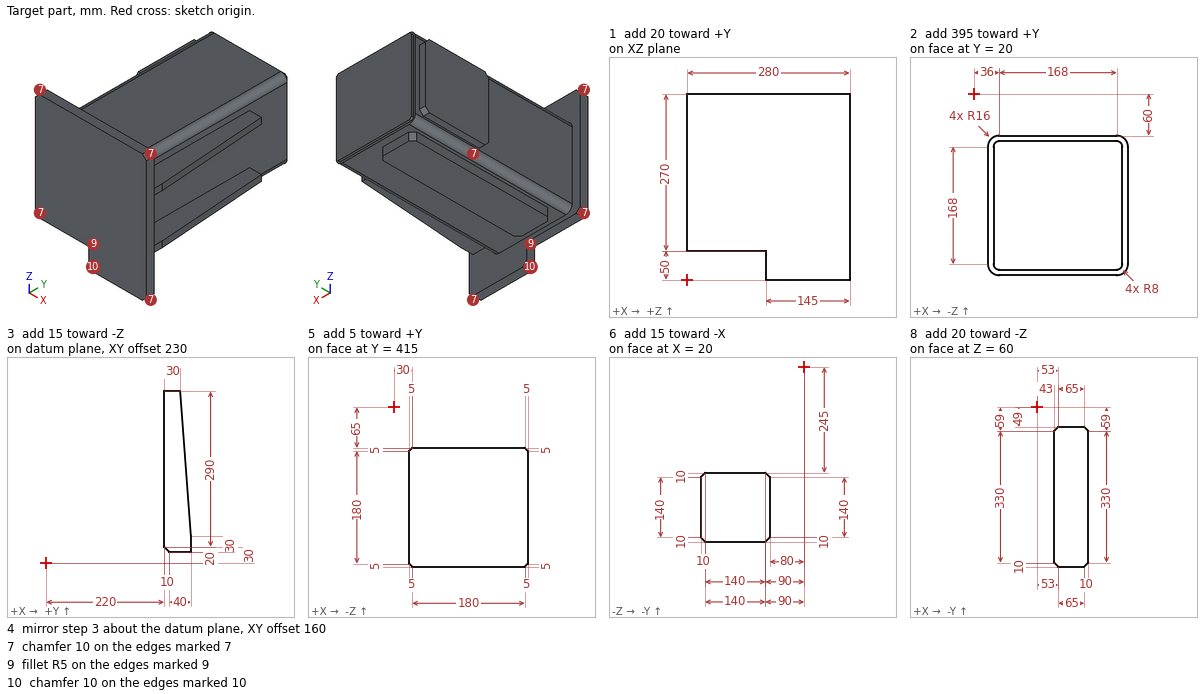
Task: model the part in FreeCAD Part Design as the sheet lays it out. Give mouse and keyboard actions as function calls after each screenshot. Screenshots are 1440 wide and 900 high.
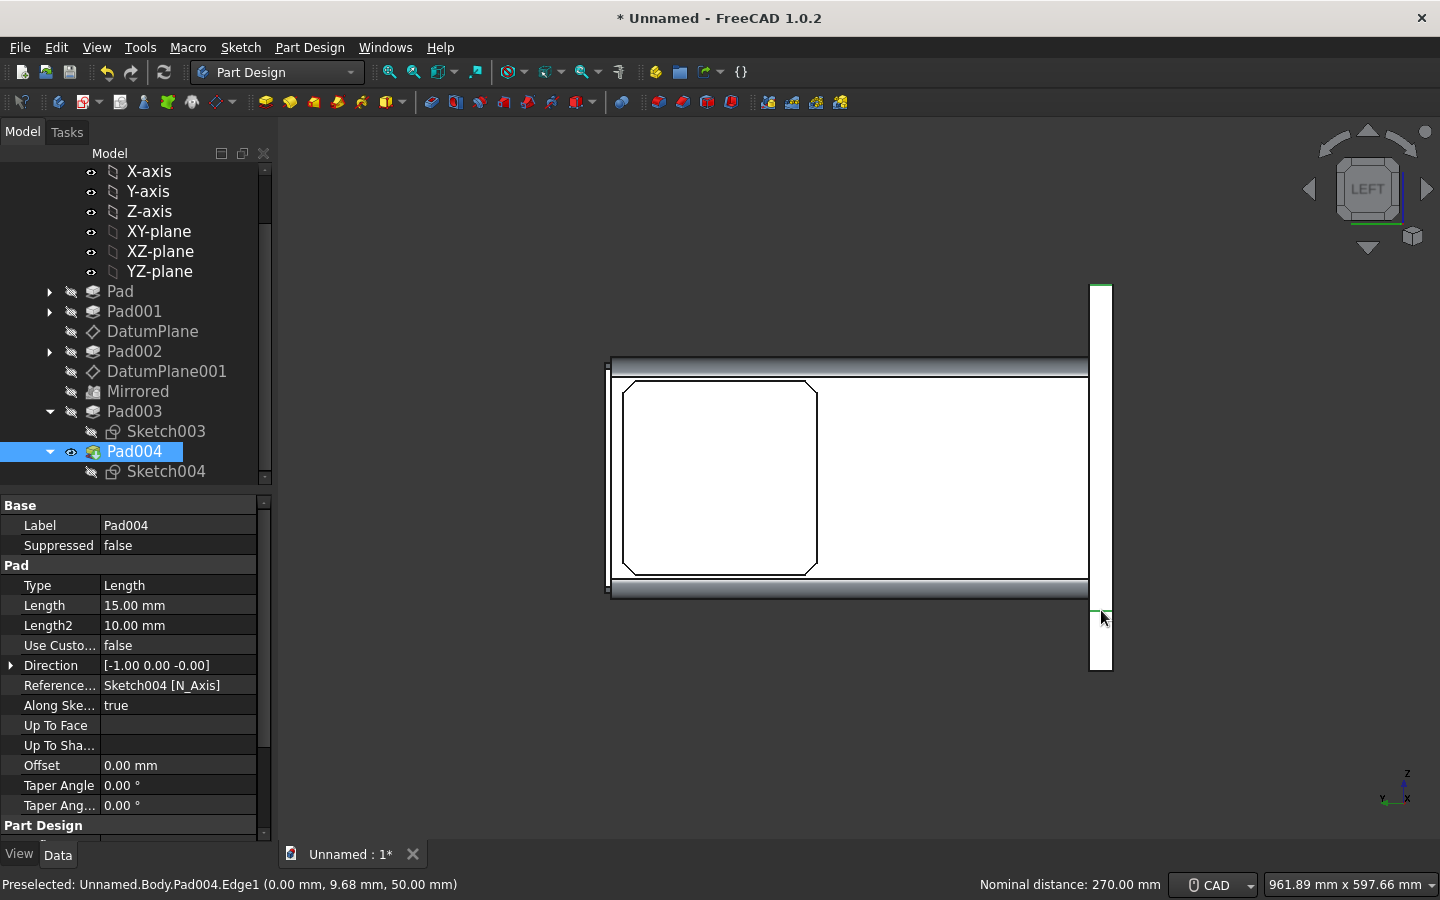
key(0)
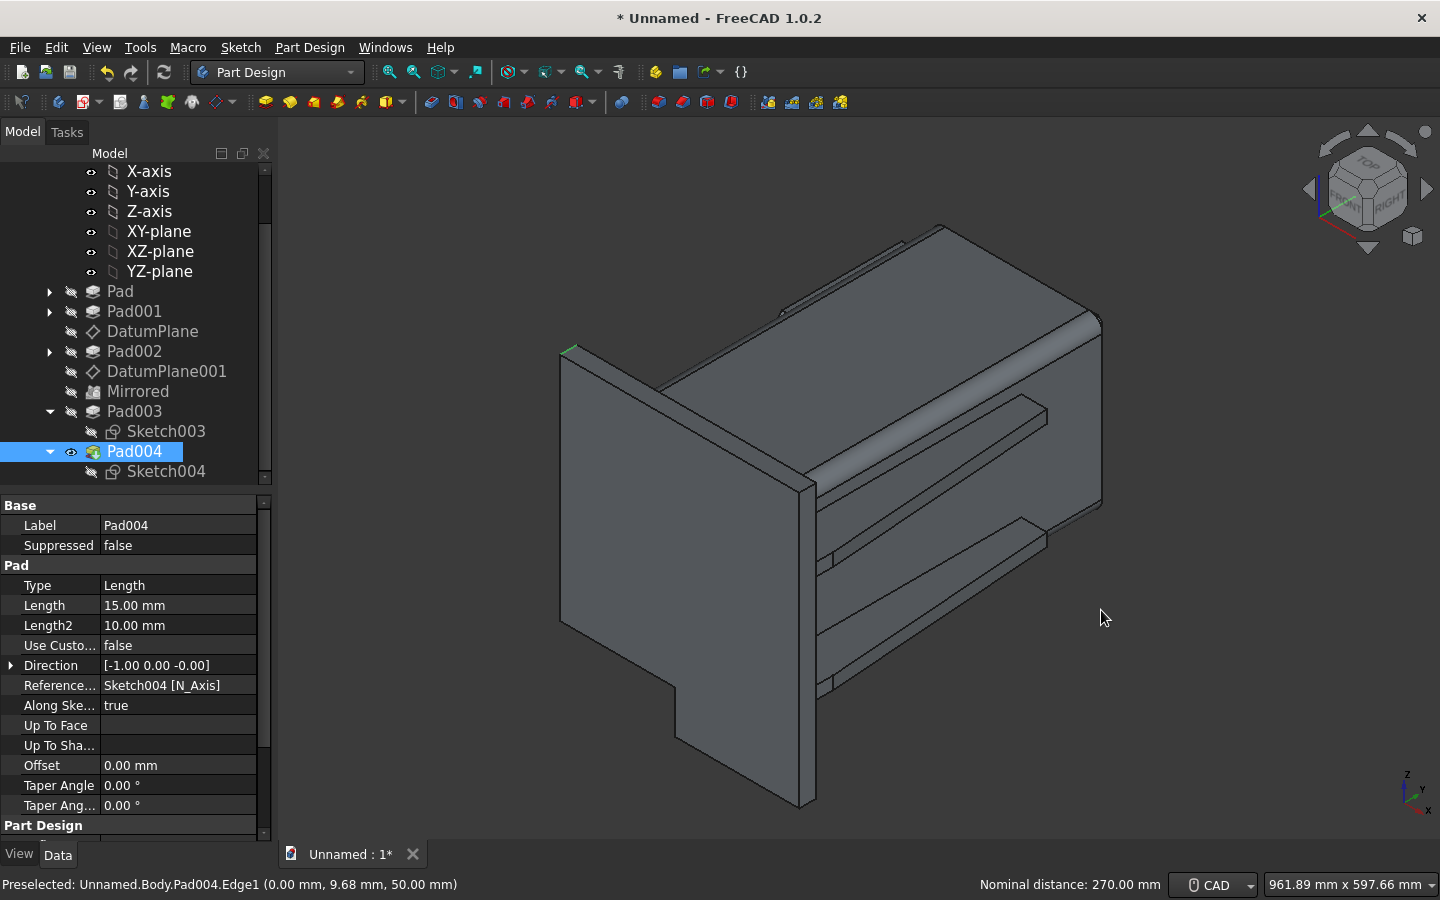
click(808, 487, ctrl)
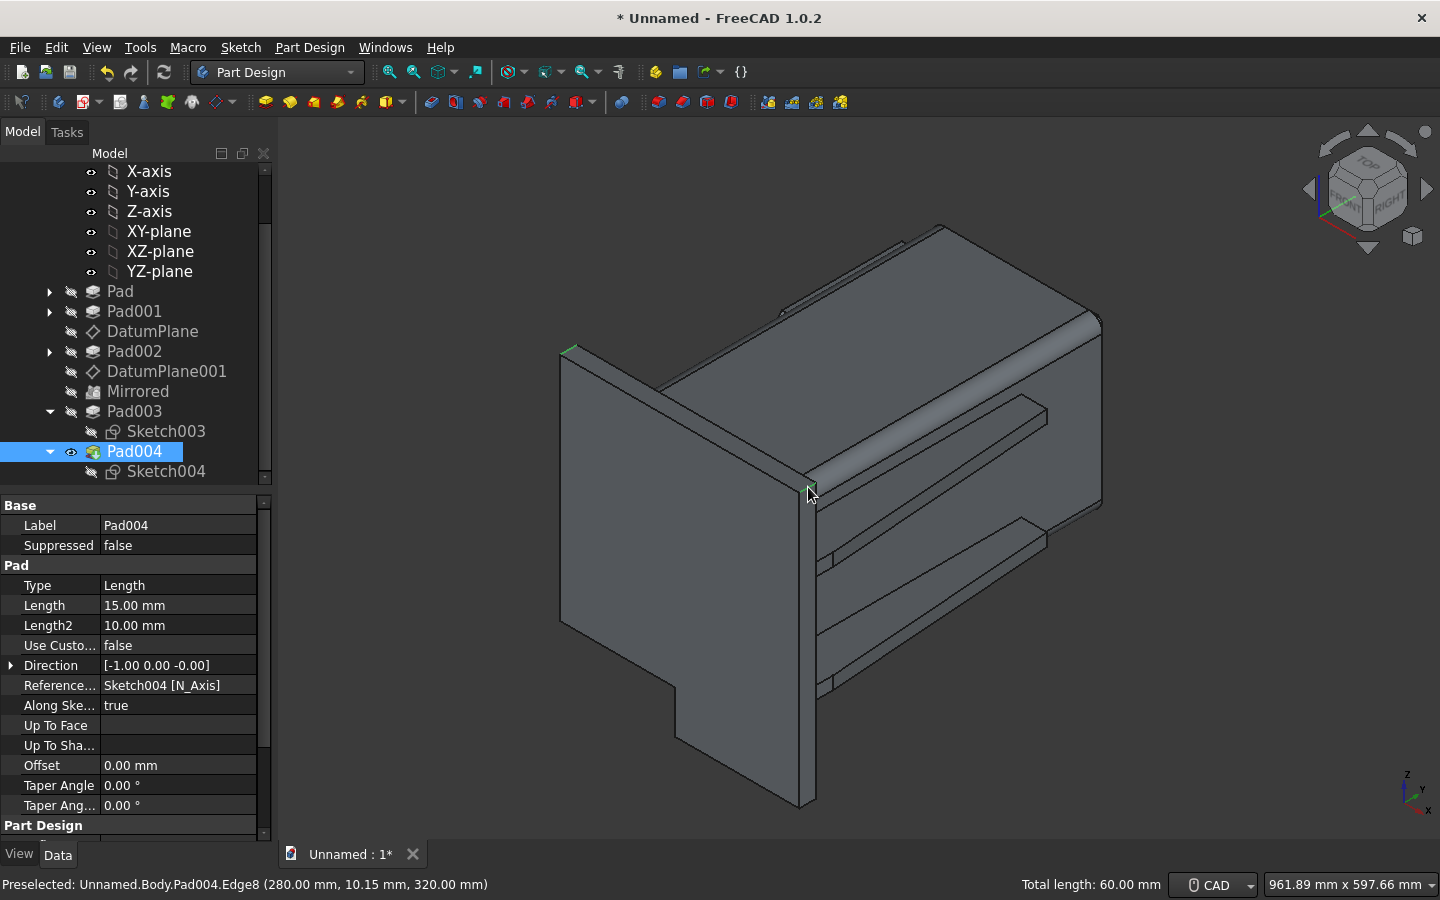
key(2)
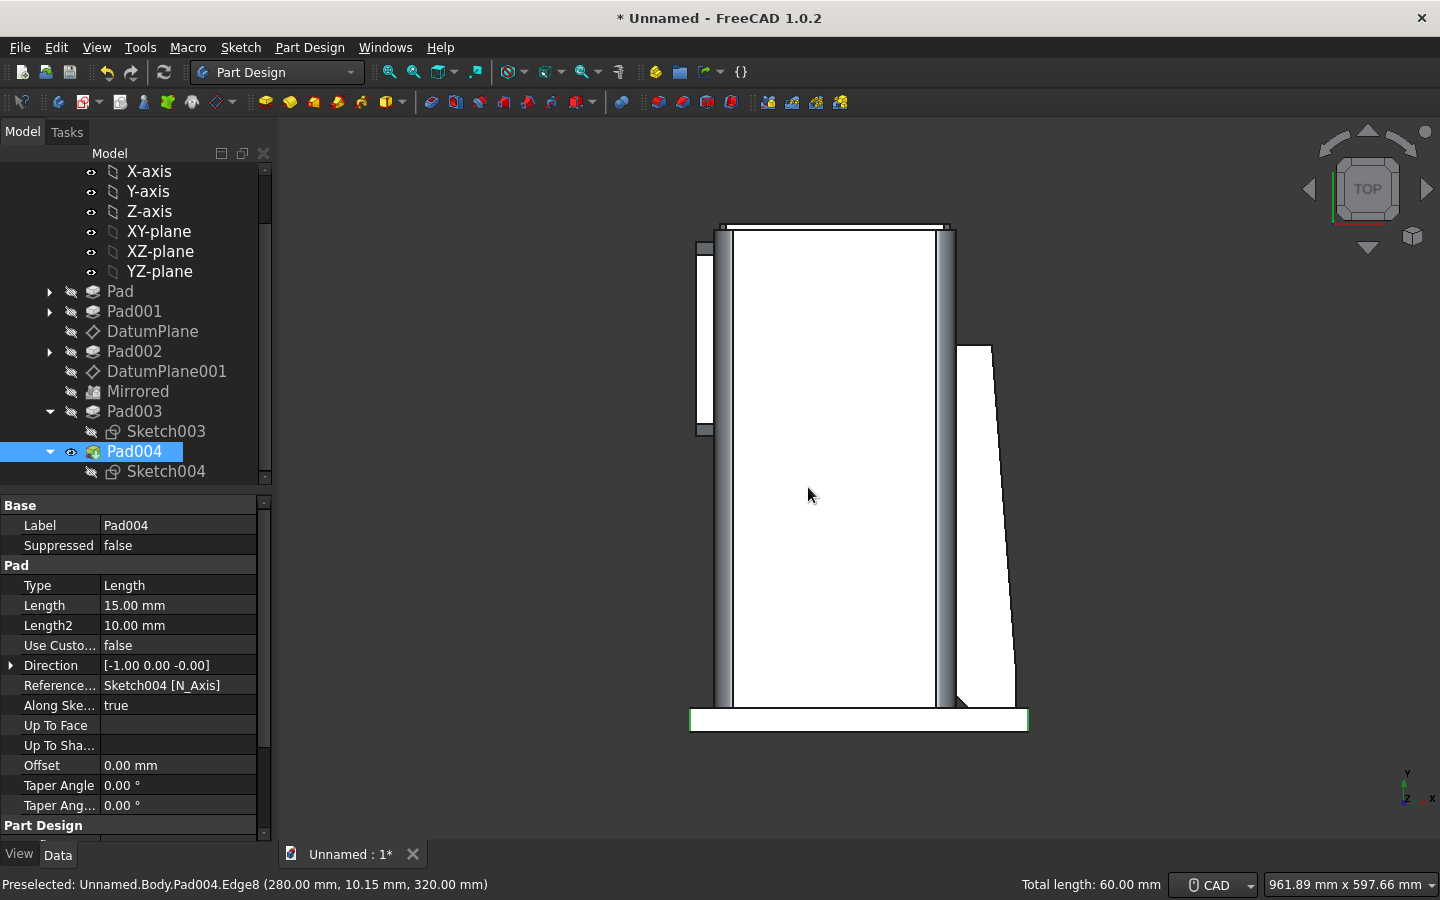
key(1)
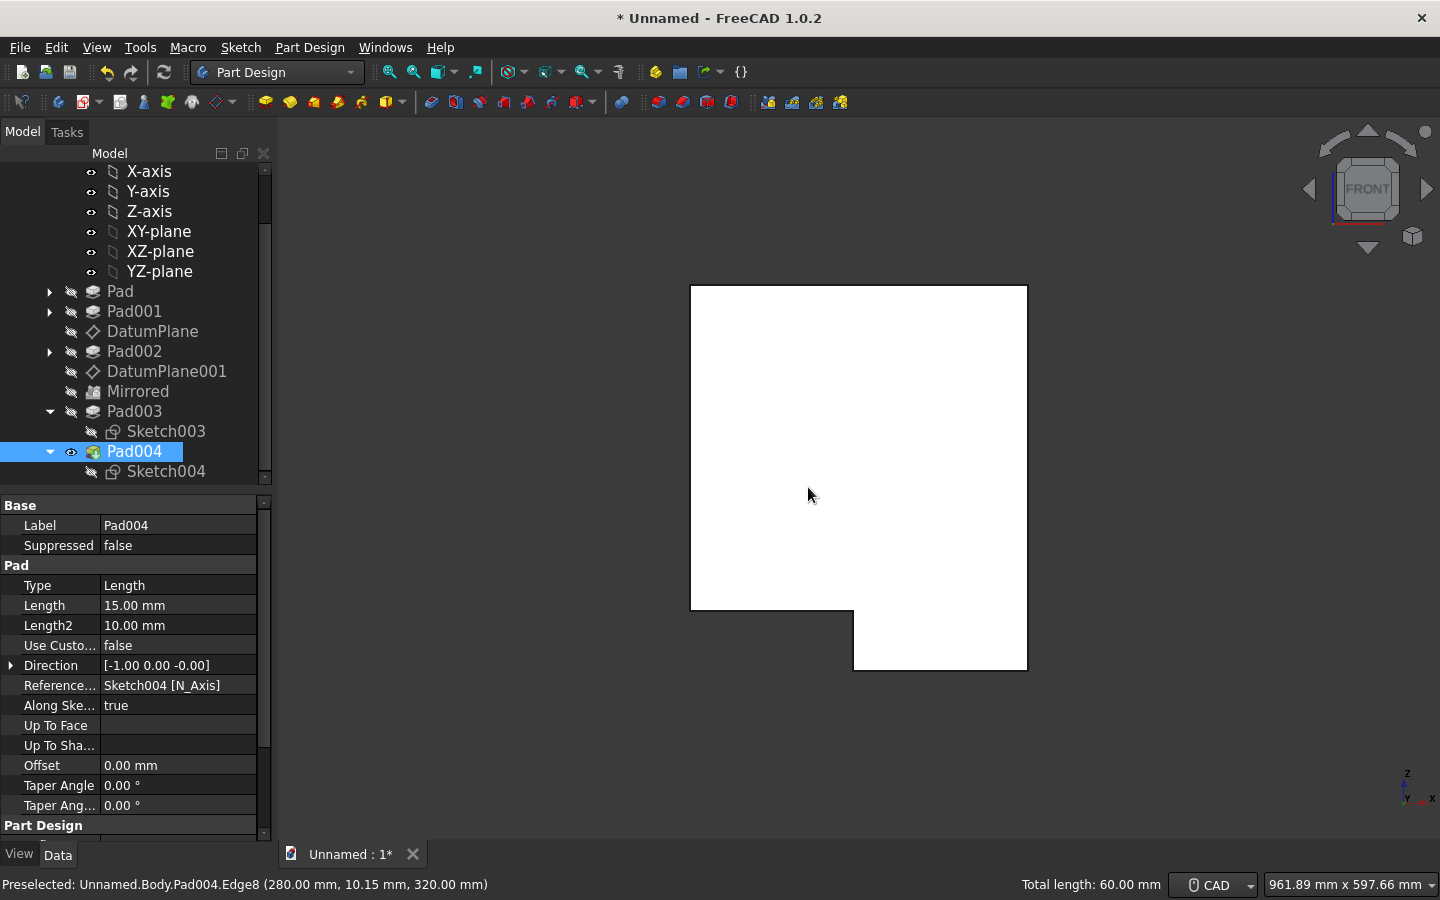
key(3)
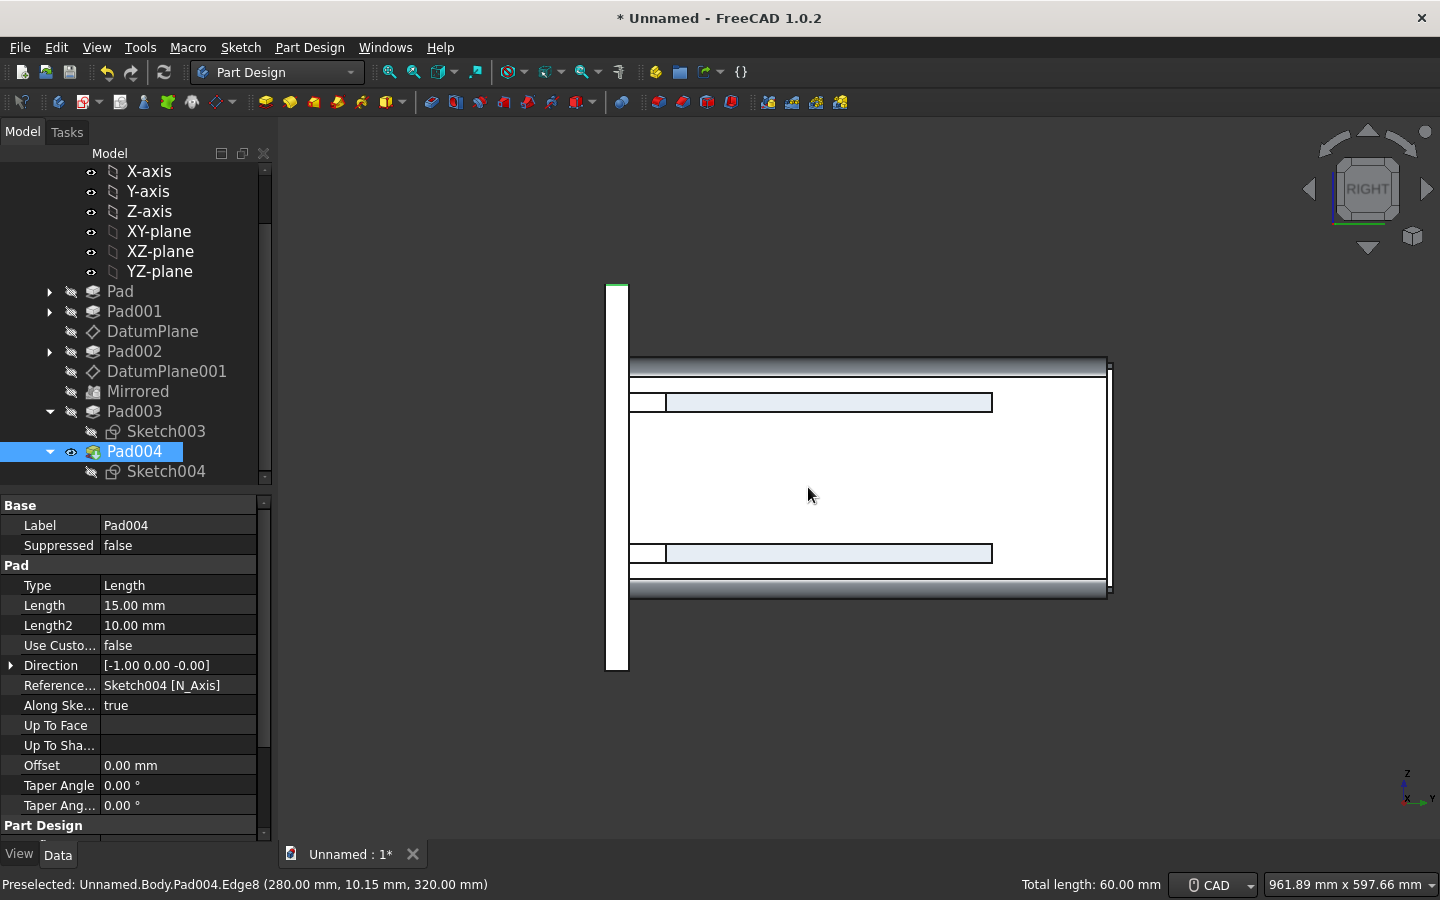
click(617, 670, ctrl)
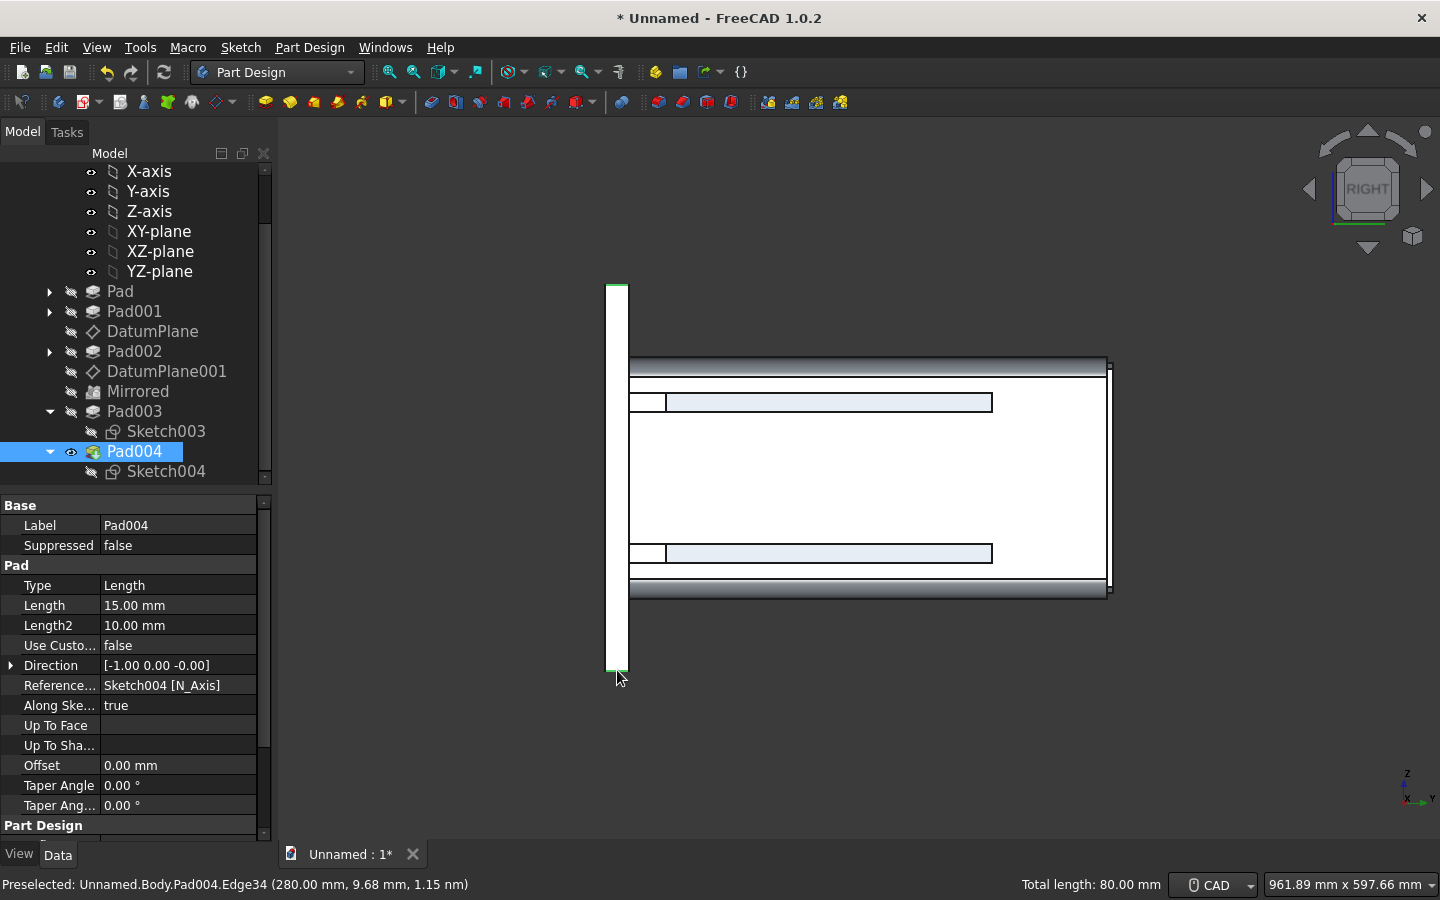
click(684, 102)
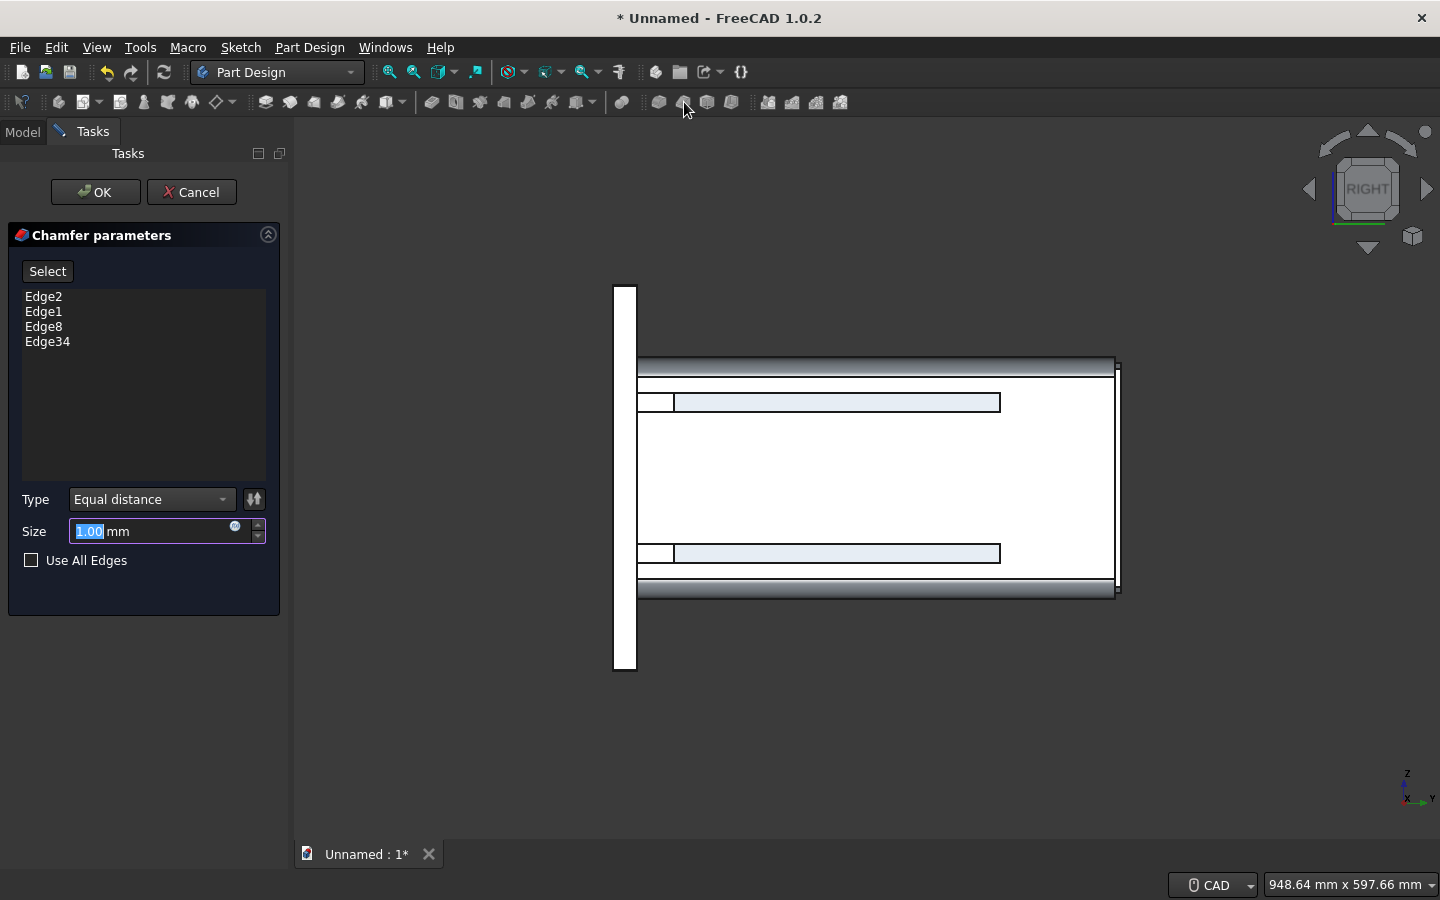
text(10)
key(Tab)